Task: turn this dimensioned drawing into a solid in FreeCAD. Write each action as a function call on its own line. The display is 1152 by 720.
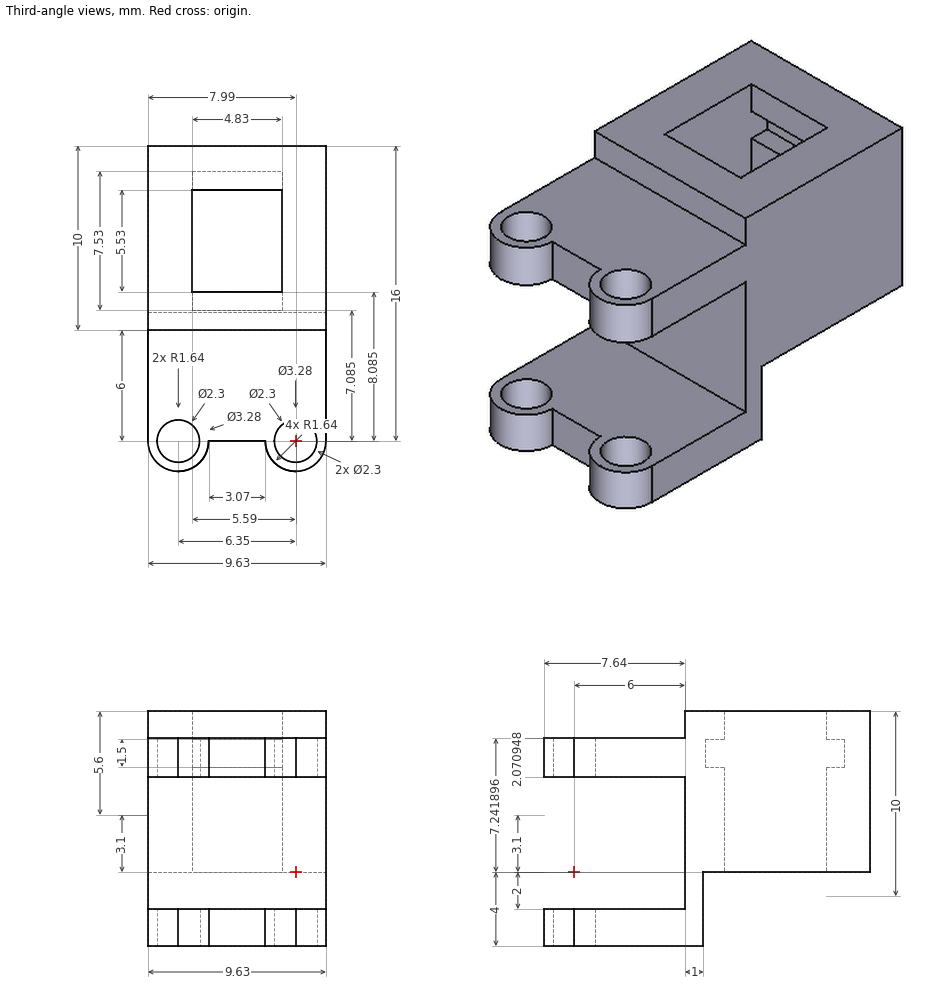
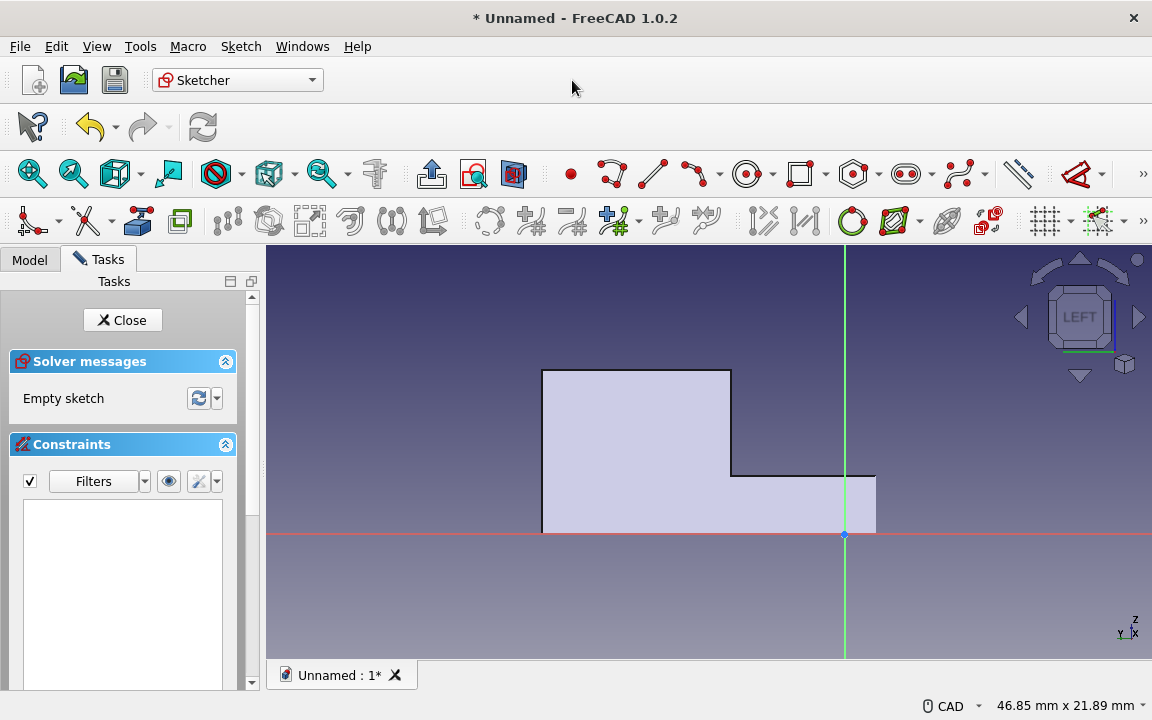
scroll(987, 631, up, 1)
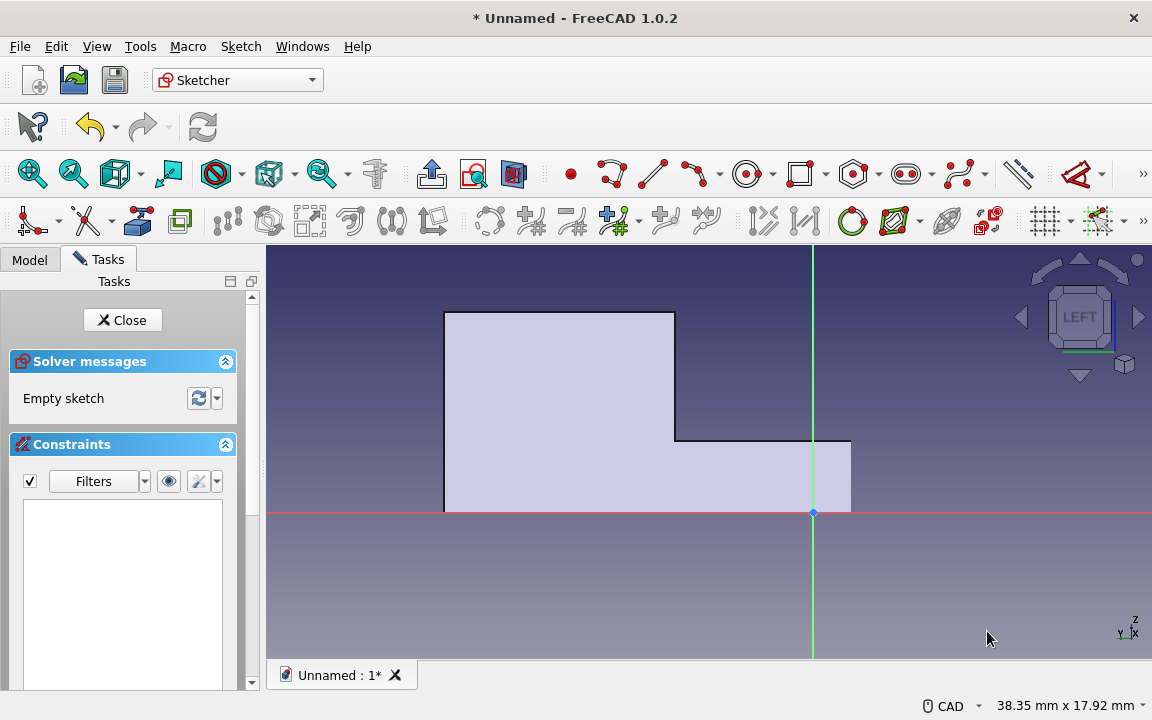
click(800, 174)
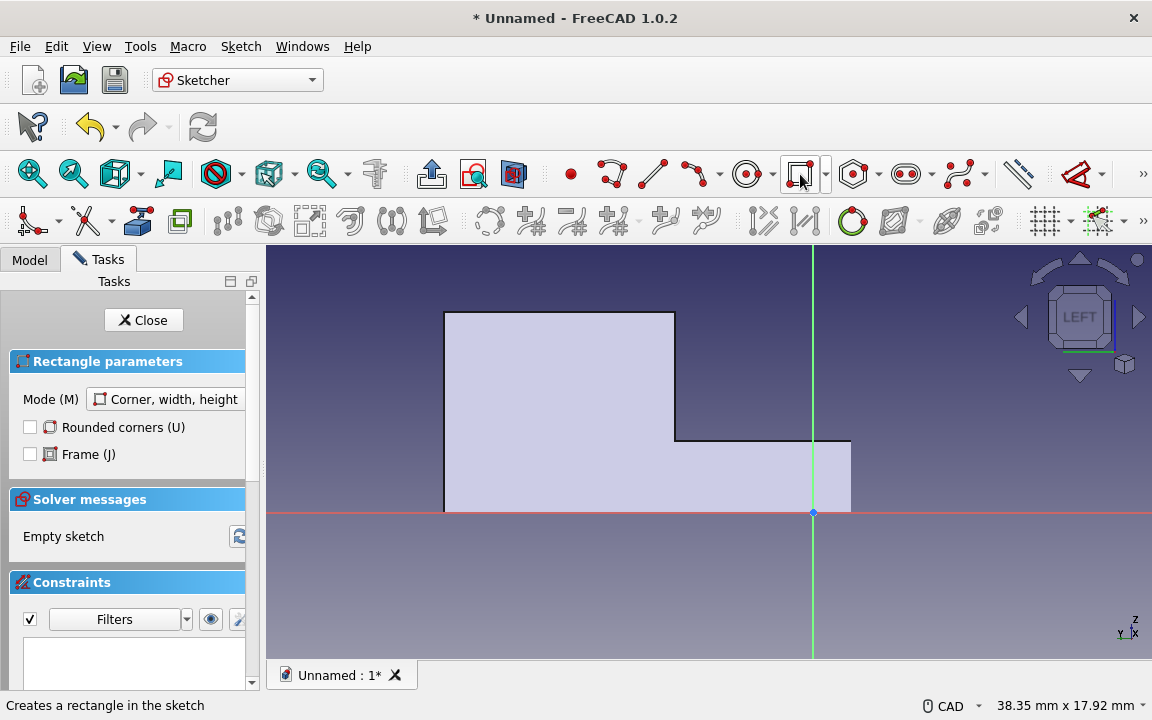
click(675, 345)
click(851, 393)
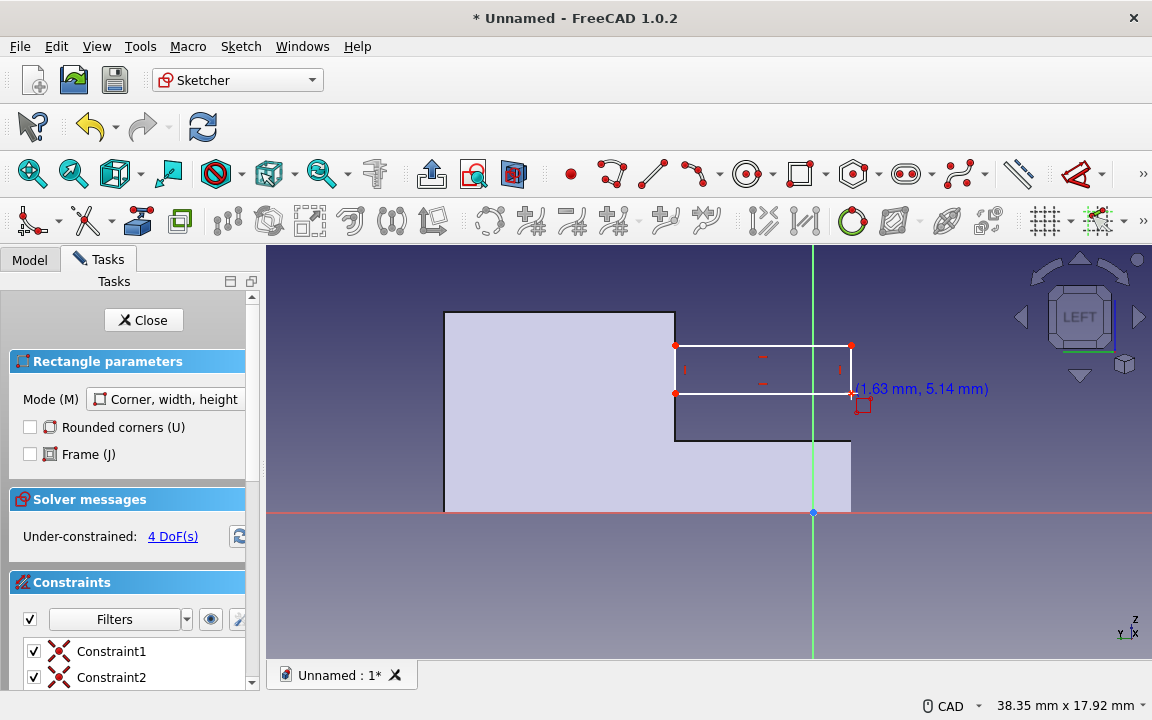
click(612, 174)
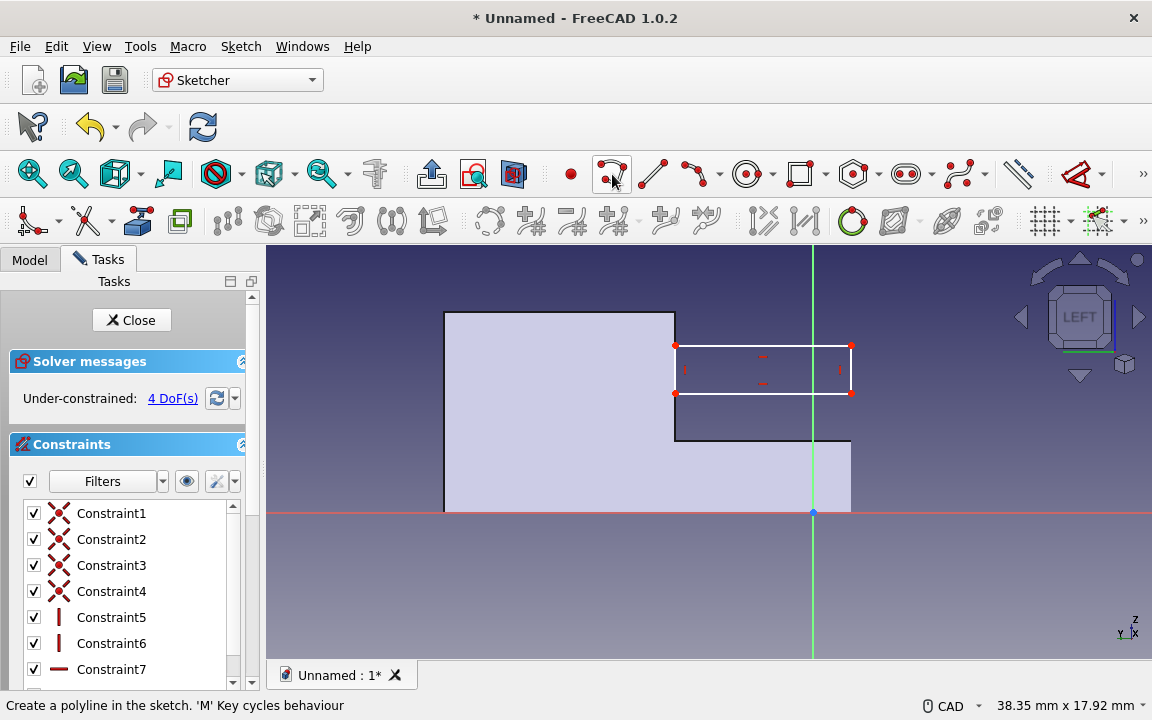
click(851, 559)
click(675, 559)
click(675, 513)
click(652, 504)
click(652, 605)
click(851, 605)
click(851, 560)
key(Escape)
key(Escape)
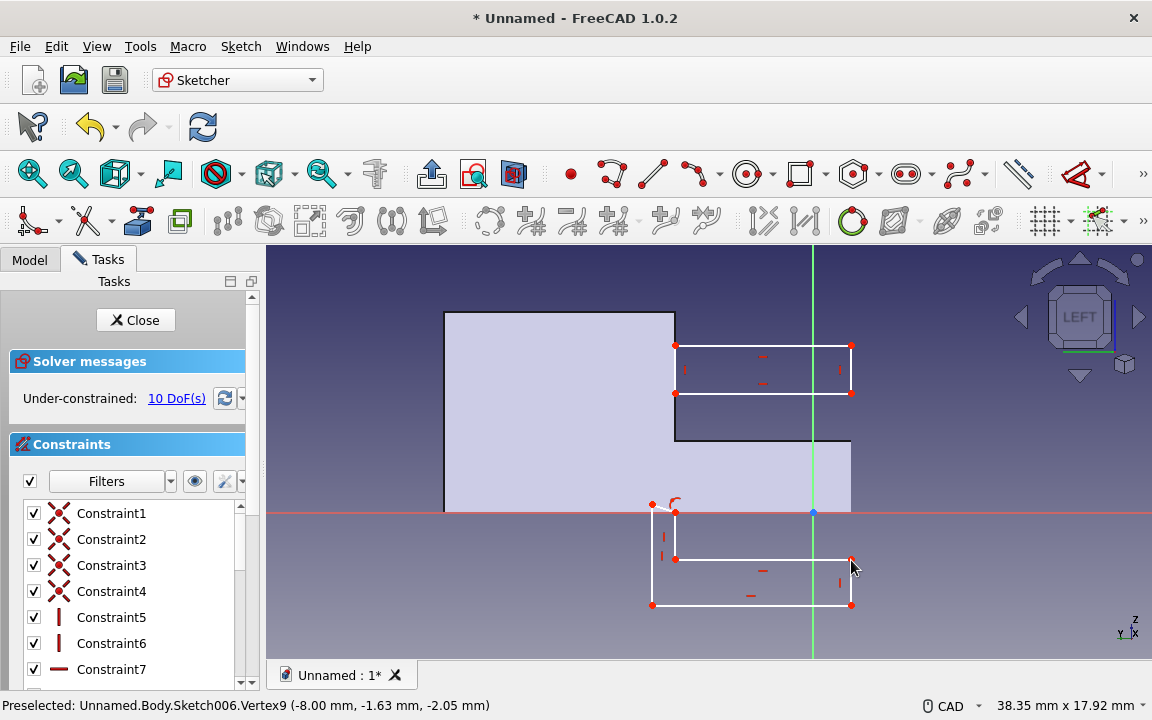
scroll(666, 510, up, 2)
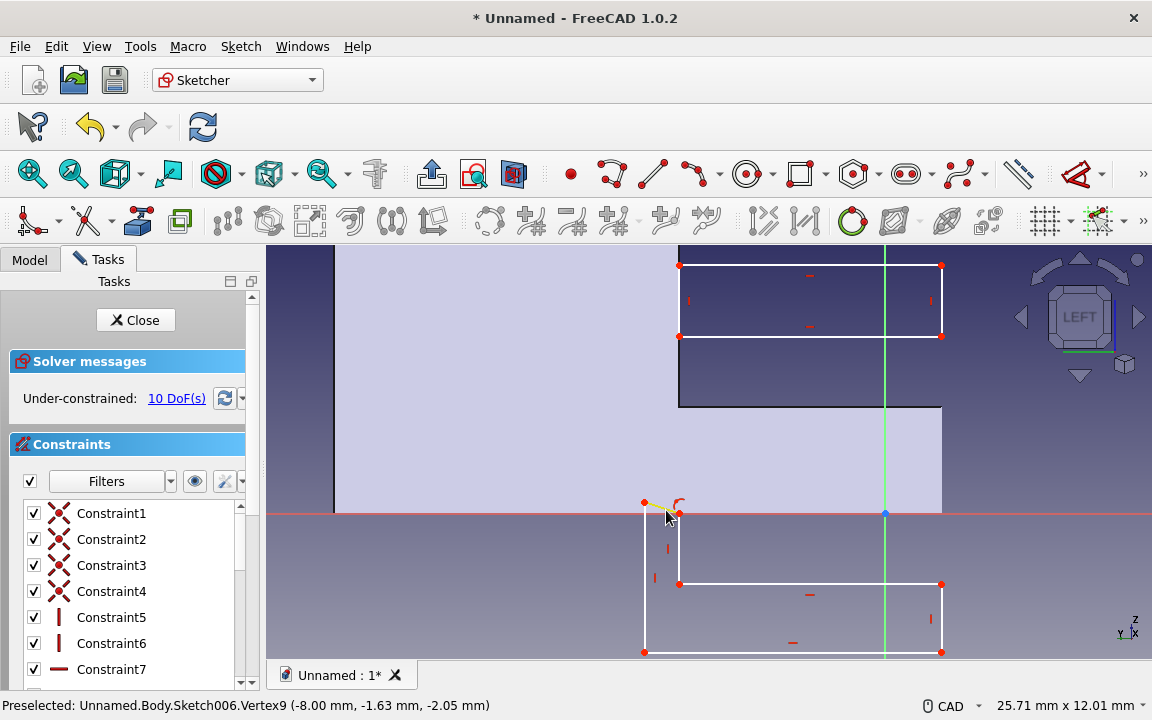
click(665, 509)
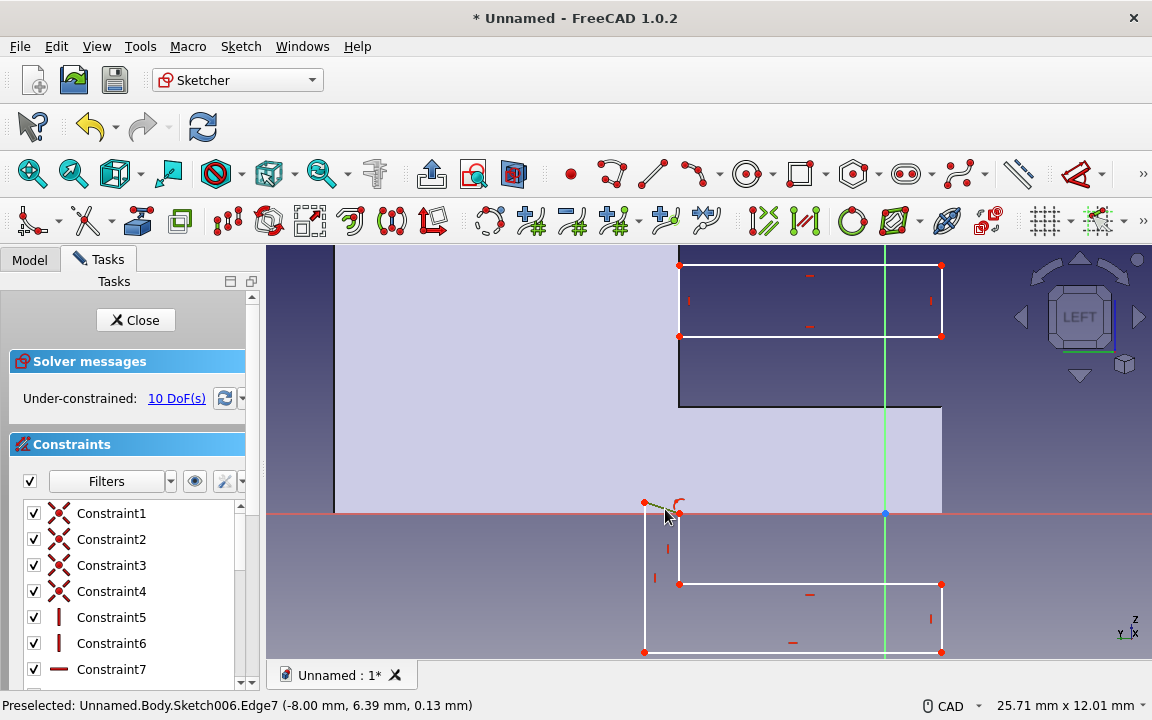
key(h)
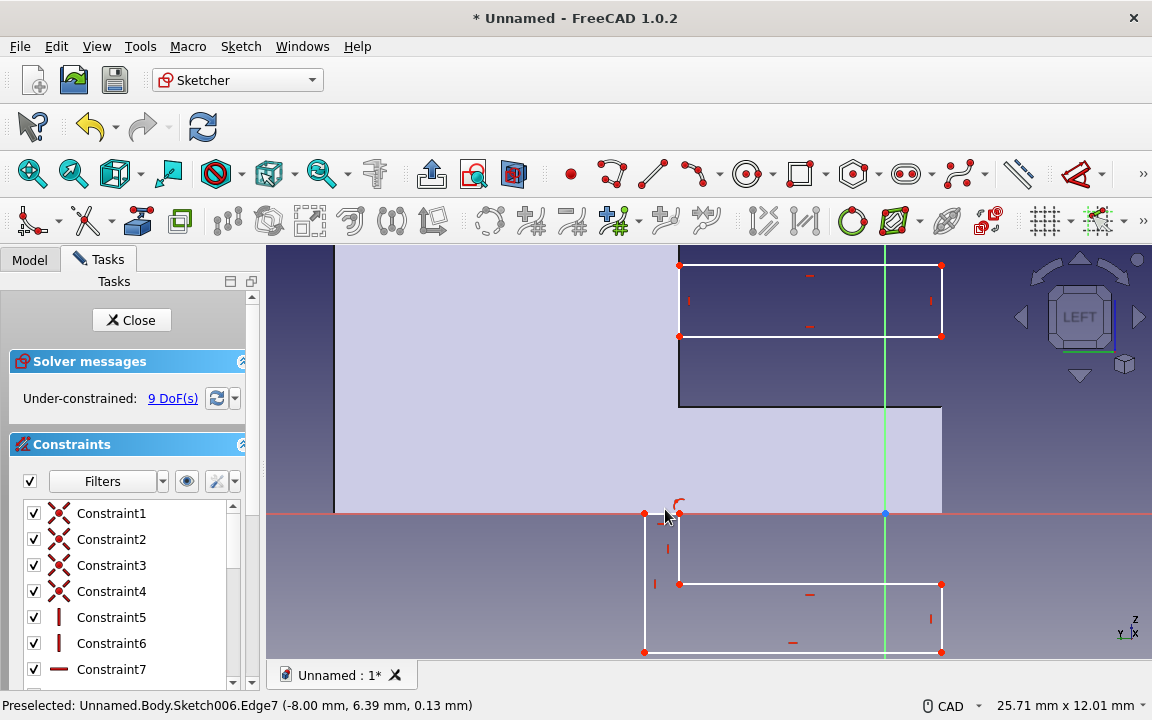
click(1076, 174)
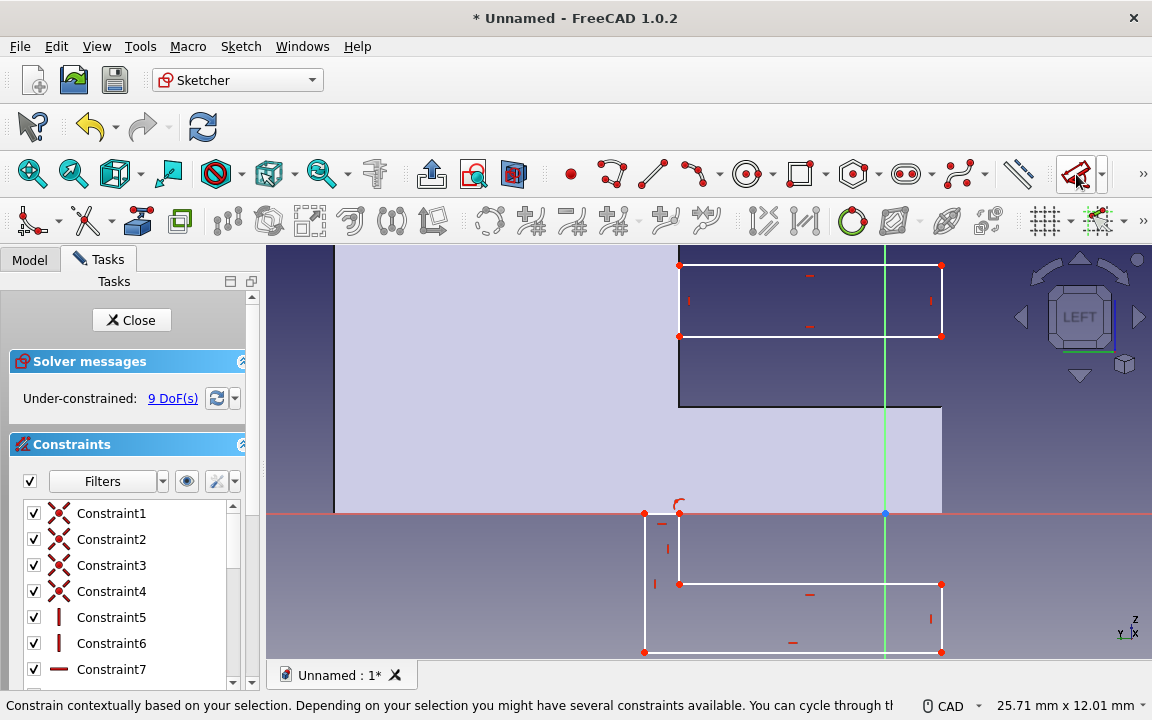
click(679, 563)
click(713, 549)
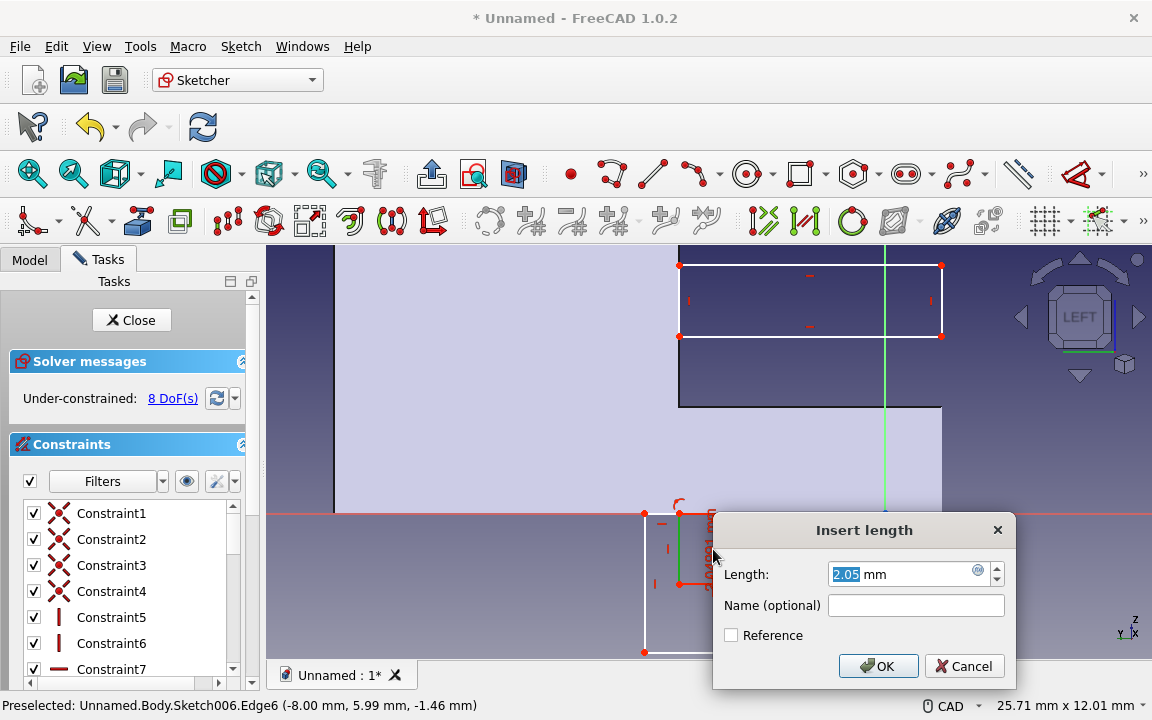
text(2)
key(Return)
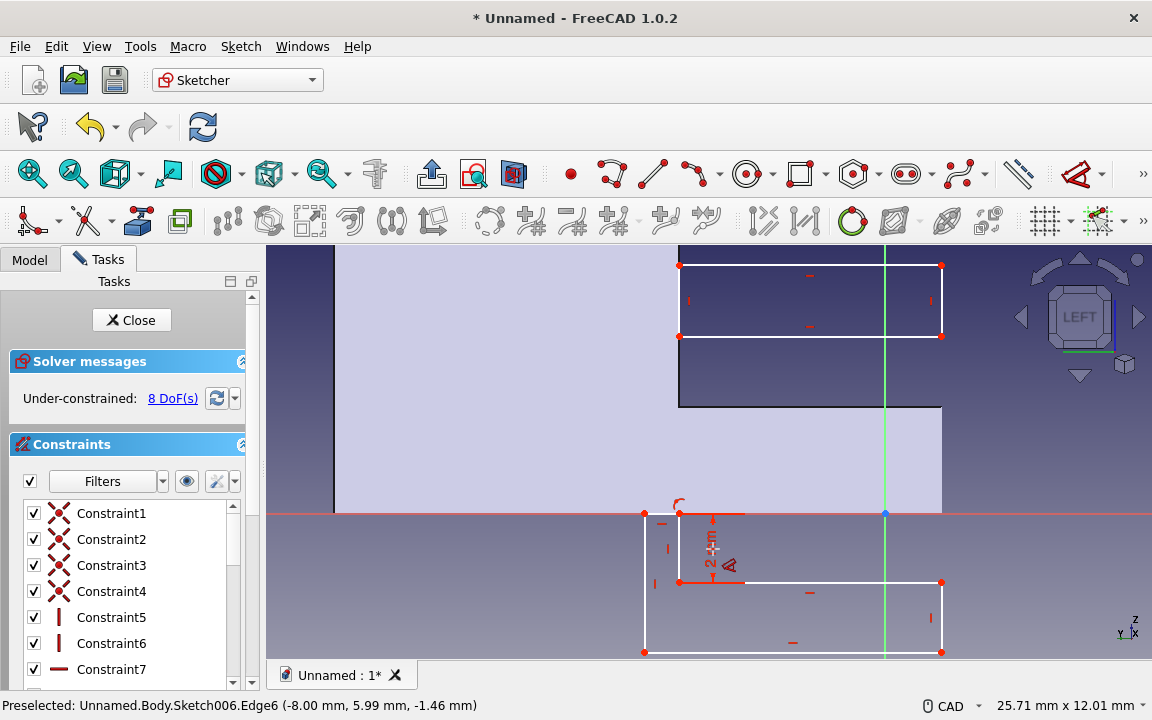
scroll(669, 514, up, 2)